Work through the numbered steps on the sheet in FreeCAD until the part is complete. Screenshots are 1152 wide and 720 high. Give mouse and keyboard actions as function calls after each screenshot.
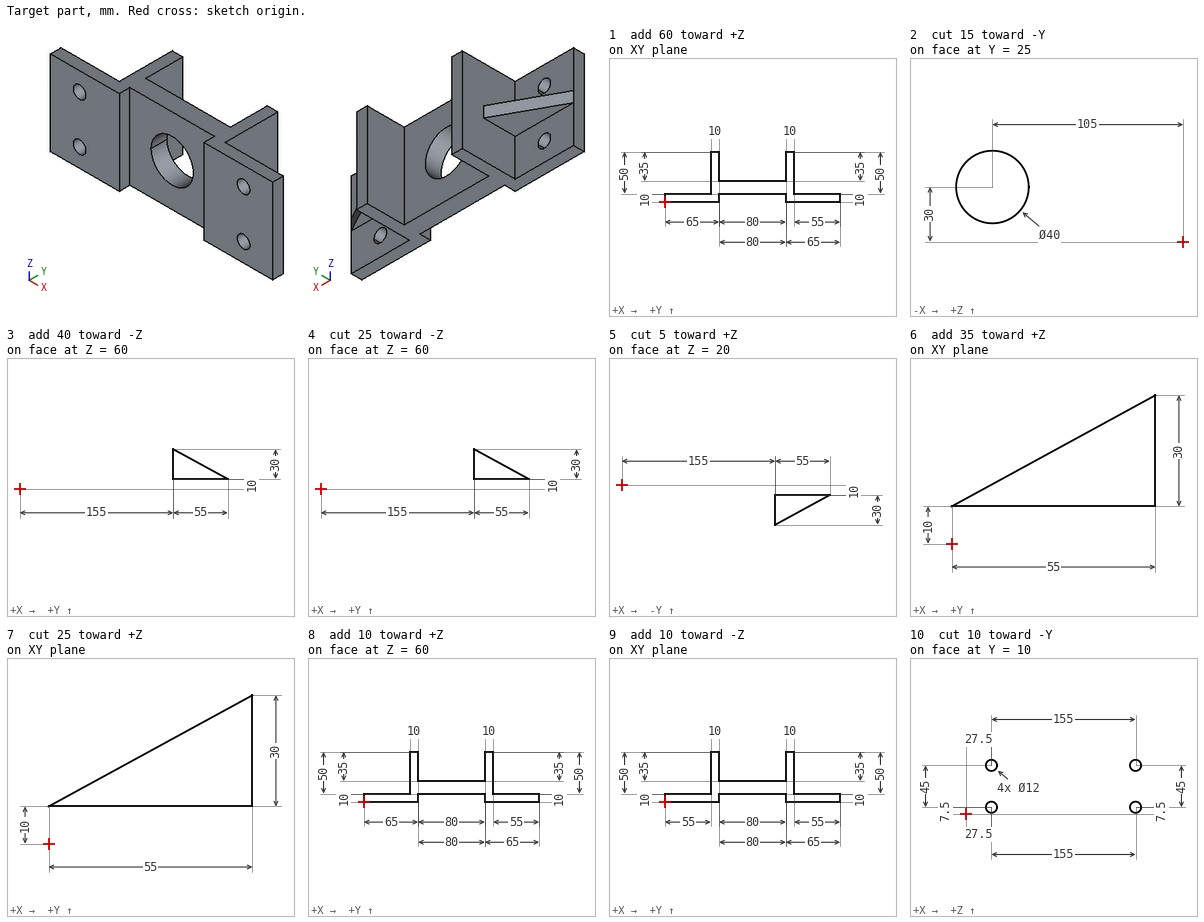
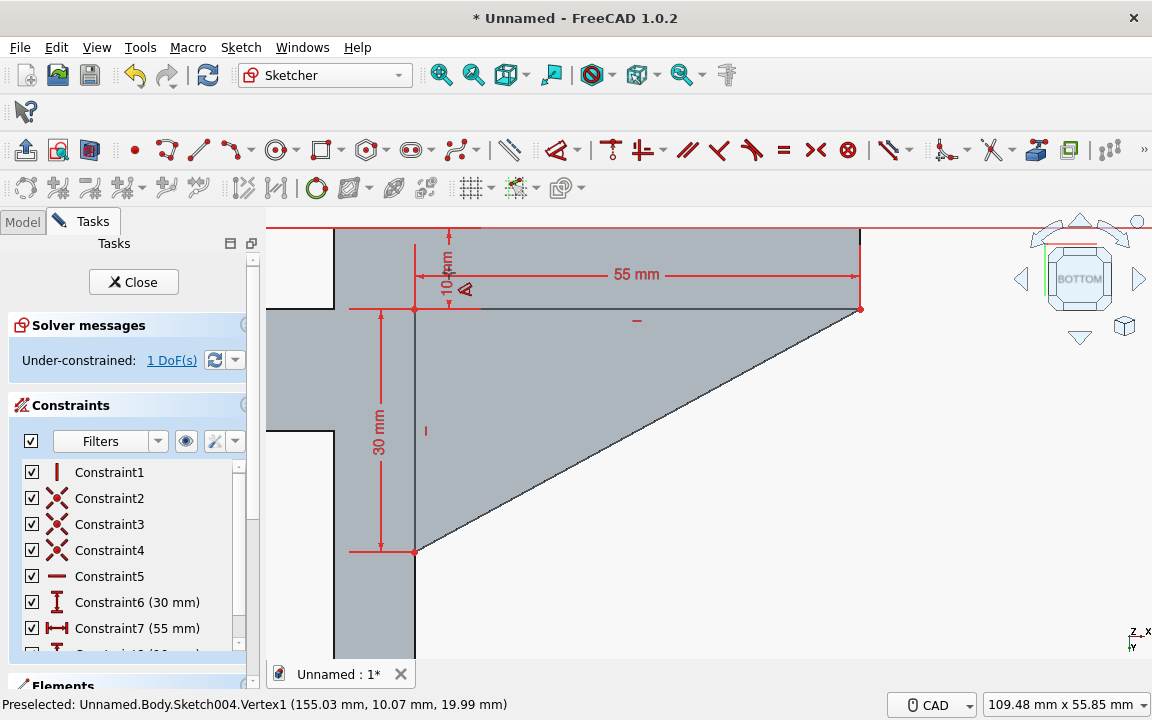
click(415, 309)
click(354, 343)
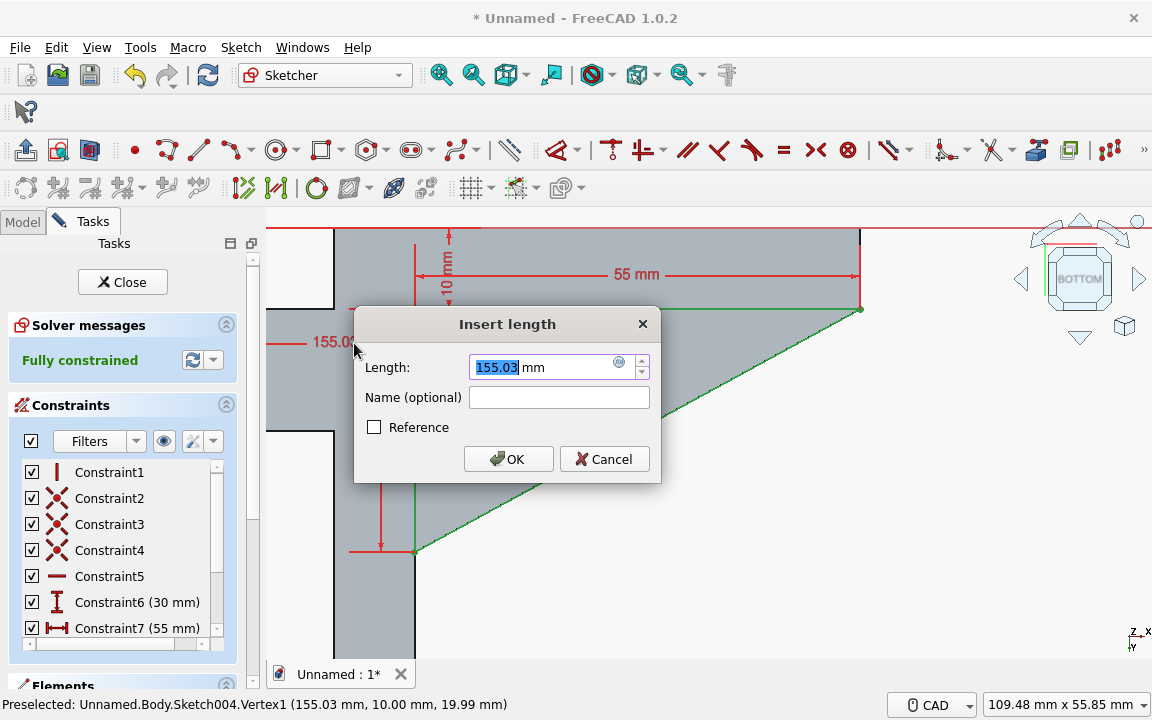
text(155)
key(Return)
key(Escape)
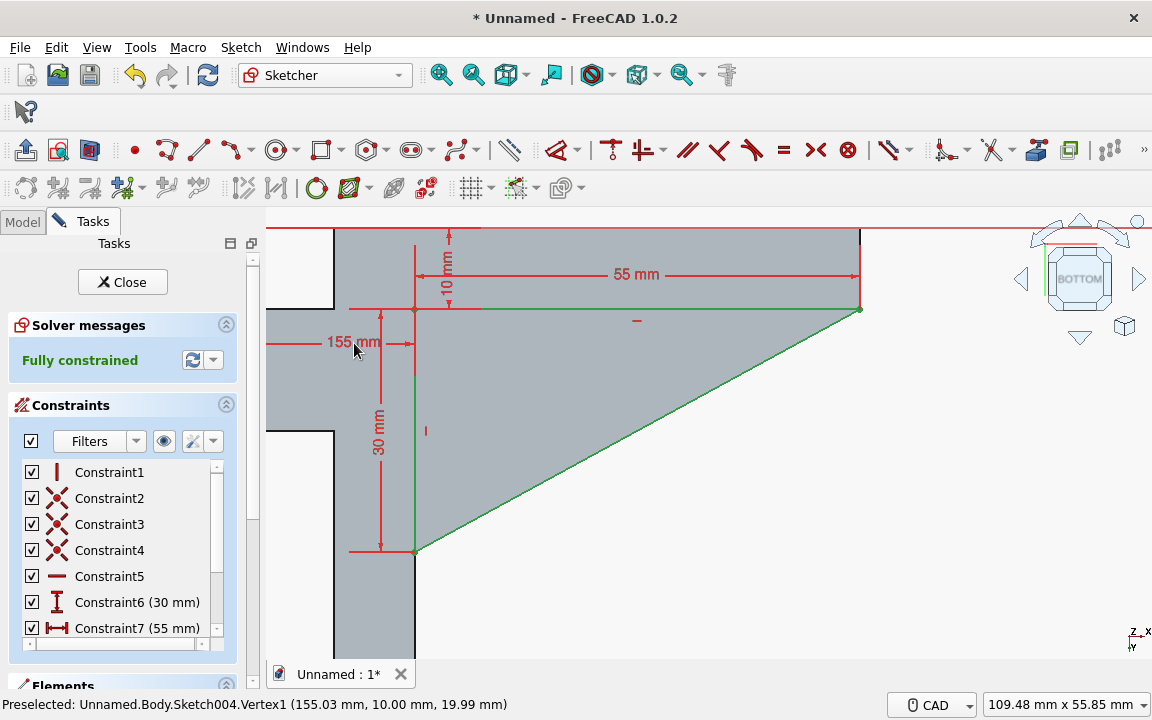
click(123, 282)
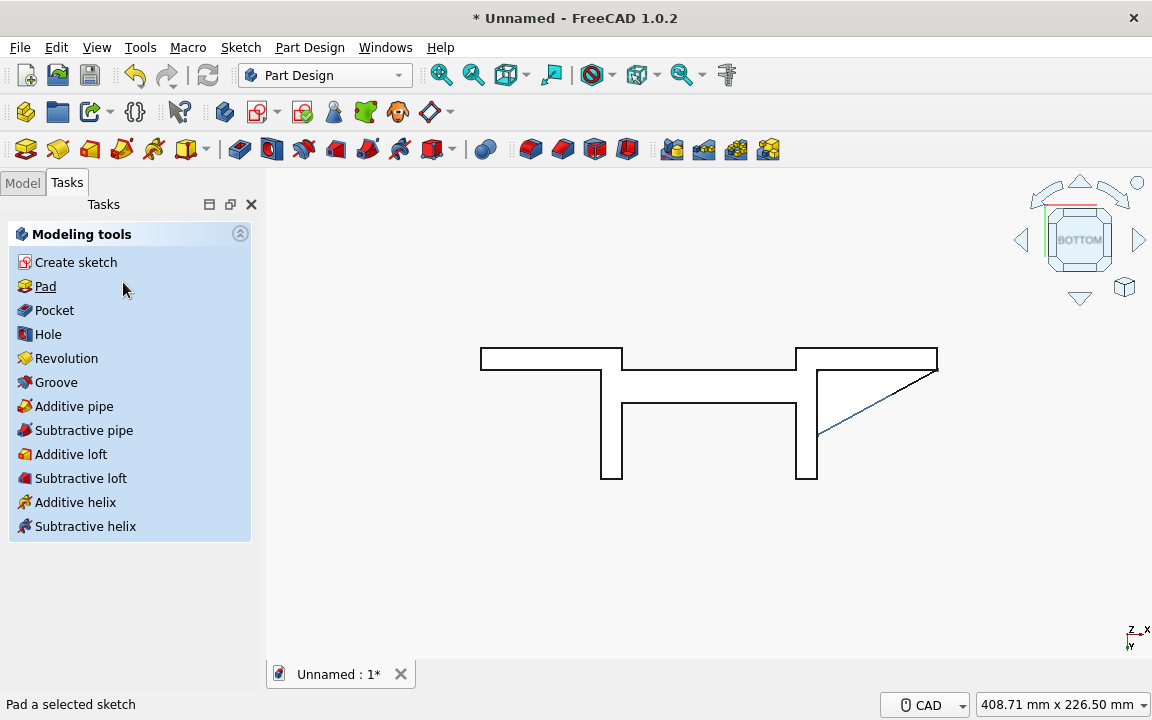
click(240, 150)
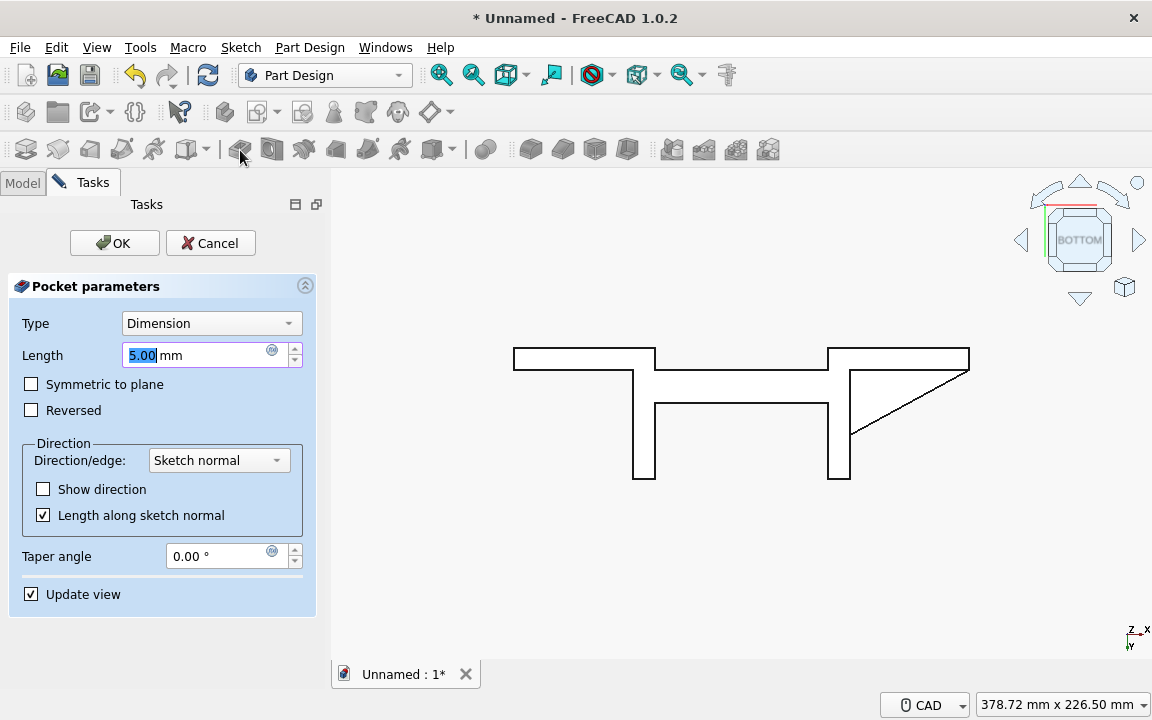
text(5)
key(Tab)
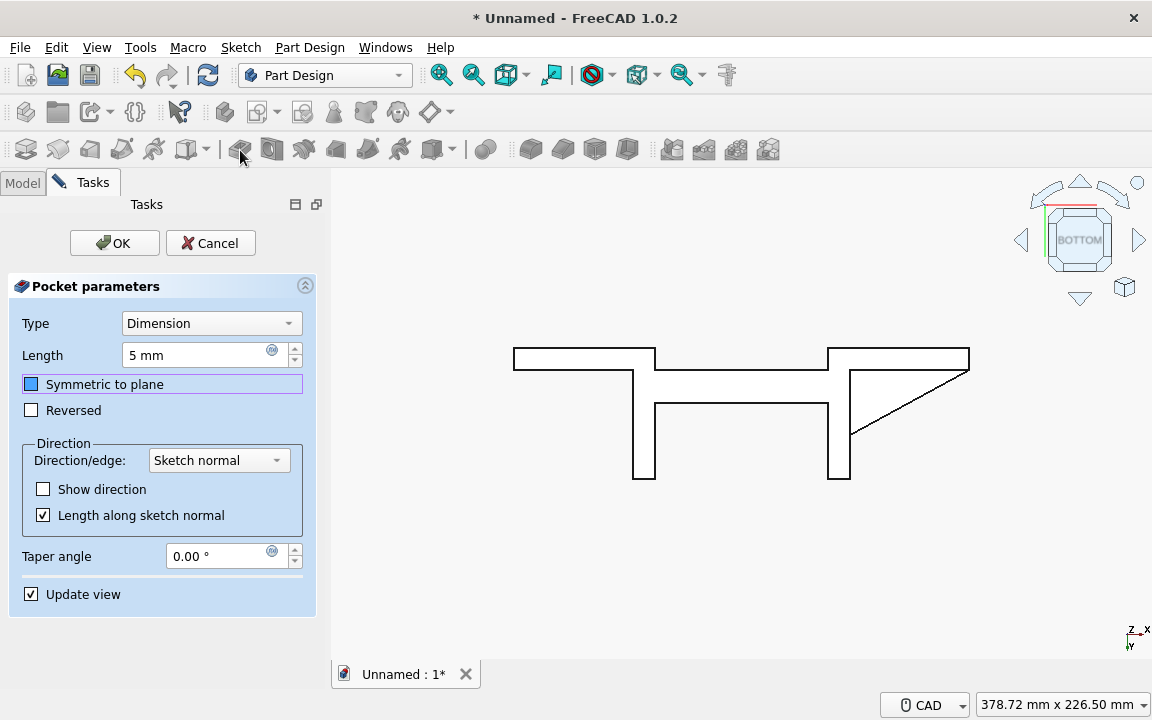
click(115, 243)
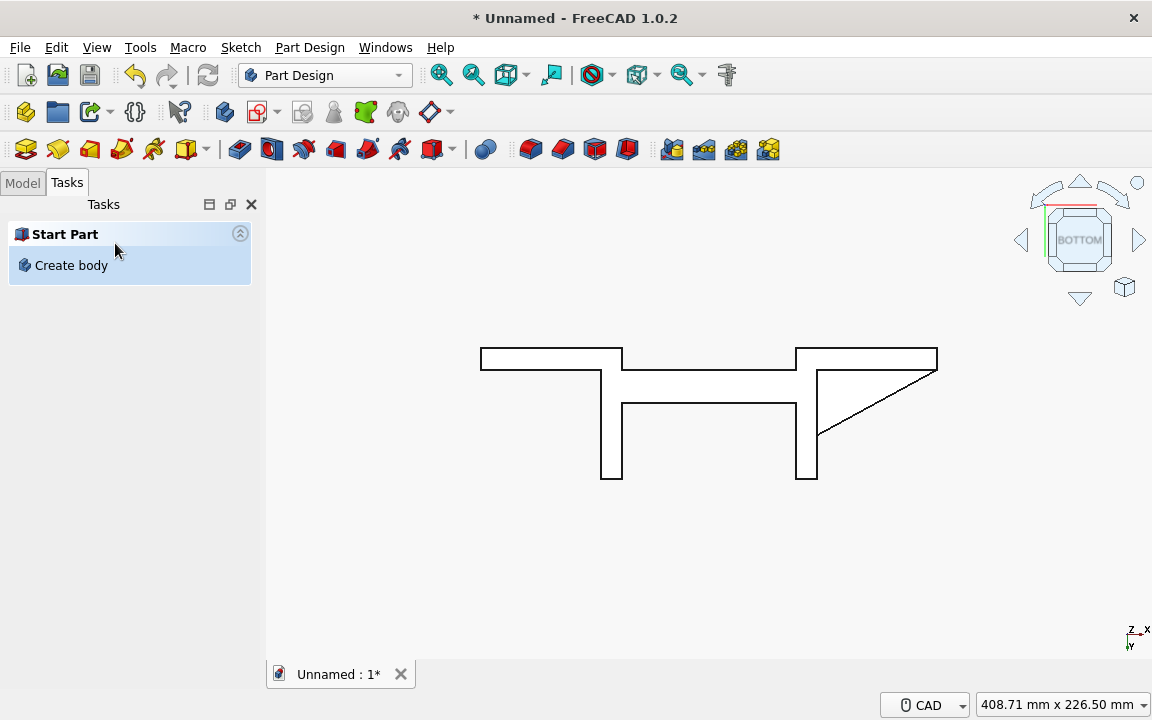
click(258, 112)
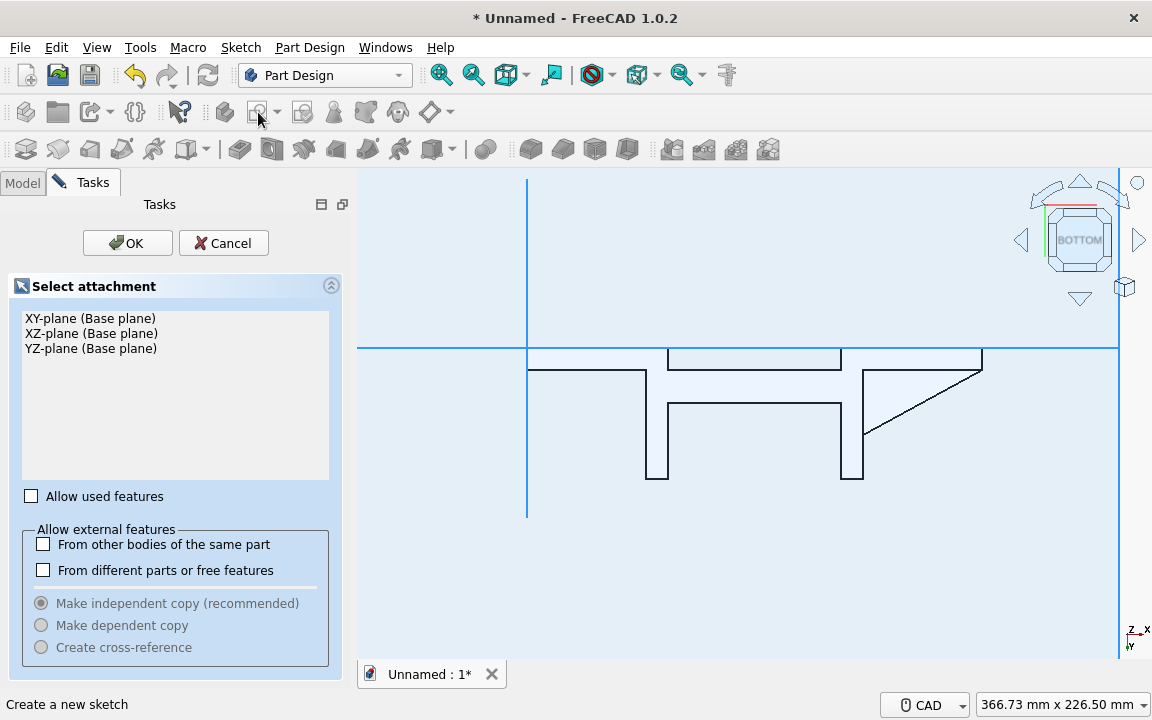
click(82, 318)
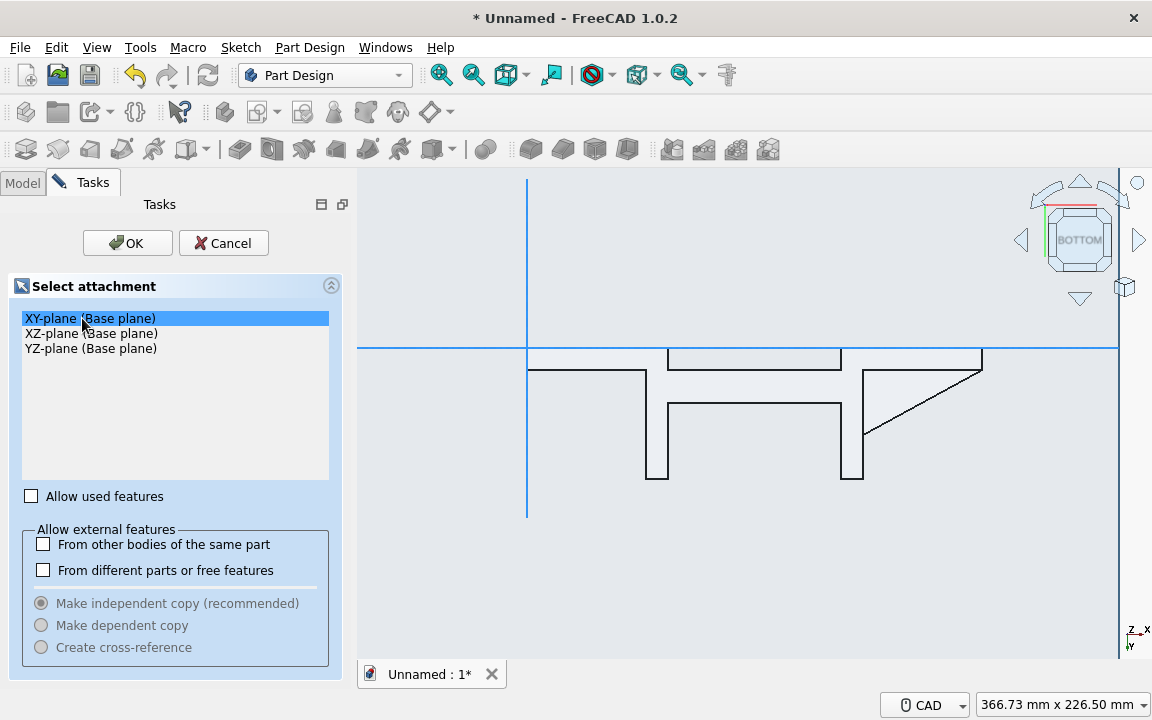
click(128, 243)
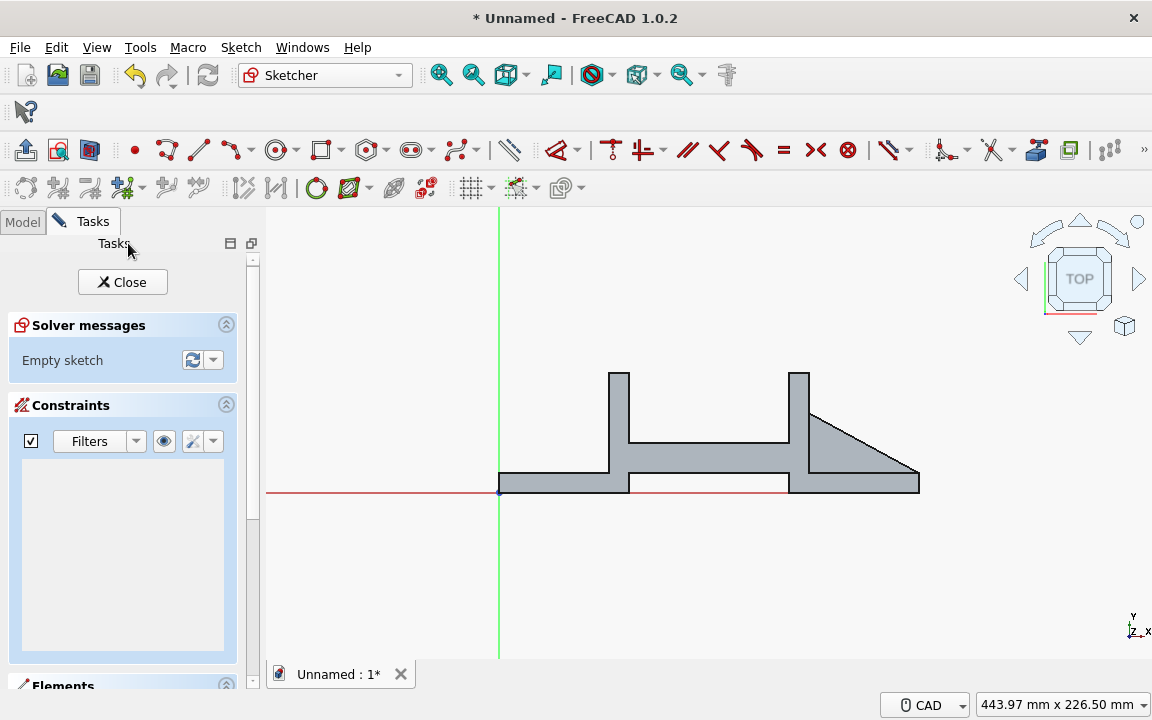
key(q)
key(s)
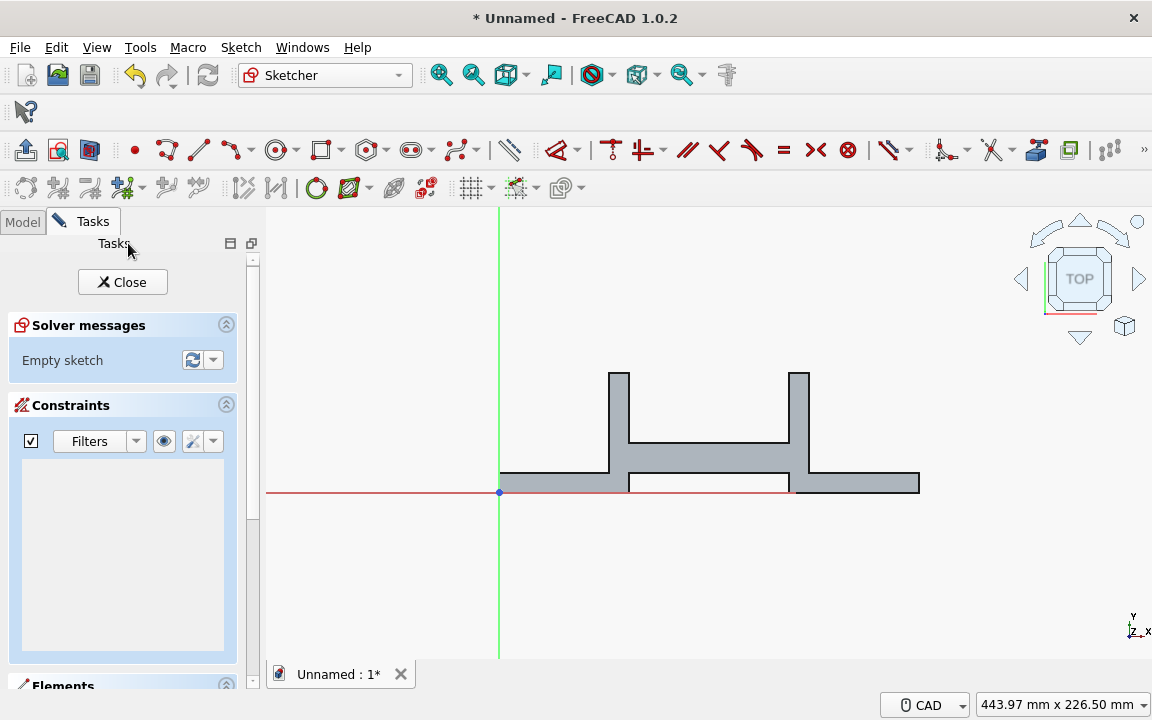
scroll(517, 462, up, 6)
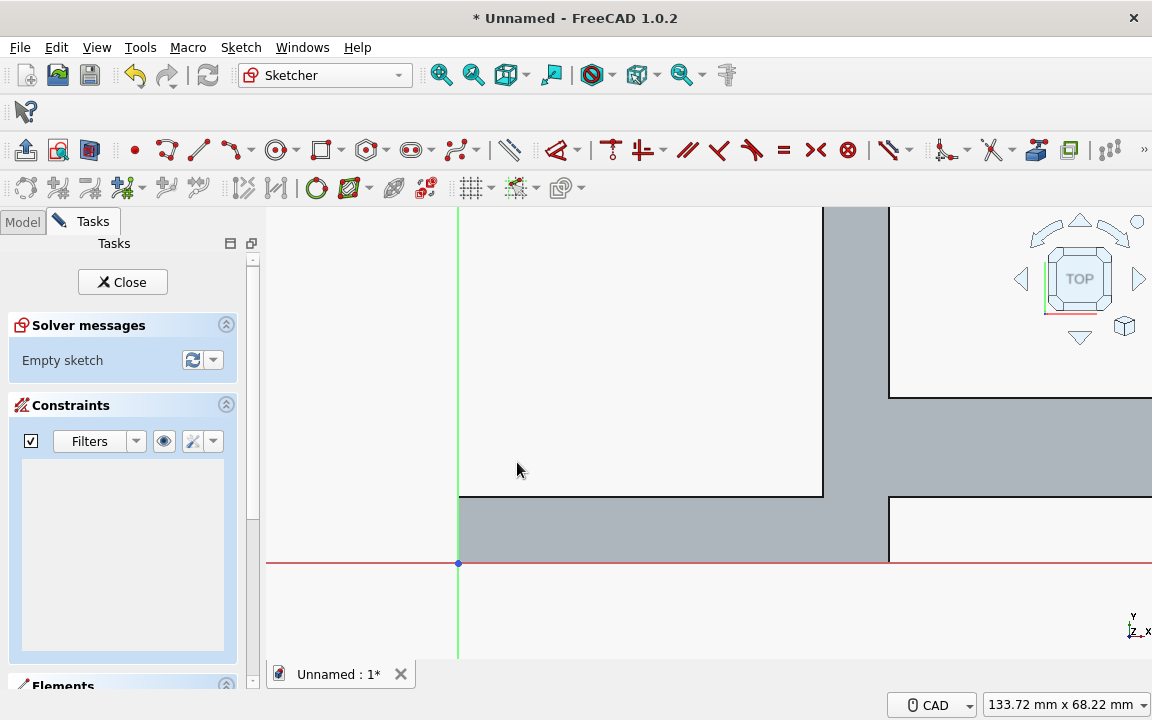
key(g)
key(m)